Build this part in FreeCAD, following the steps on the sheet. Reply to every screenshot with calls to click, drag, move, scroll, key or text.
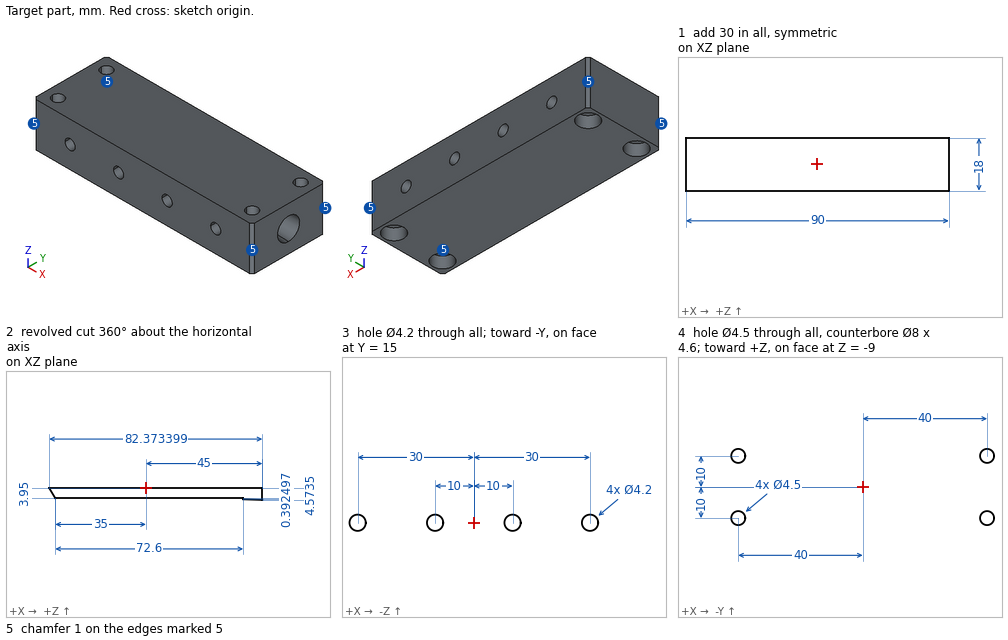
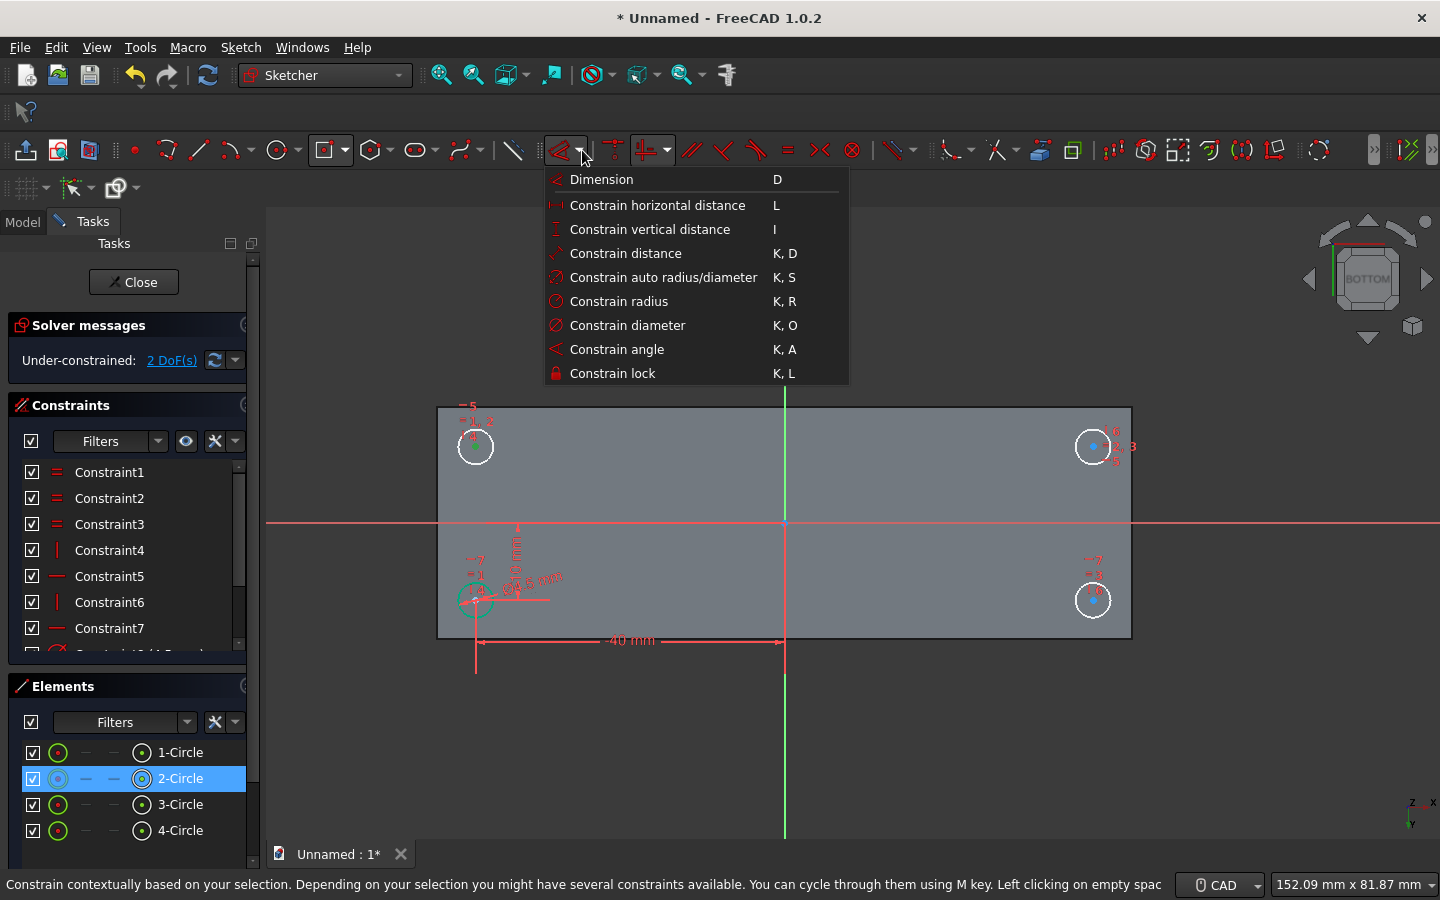
click(697, 229)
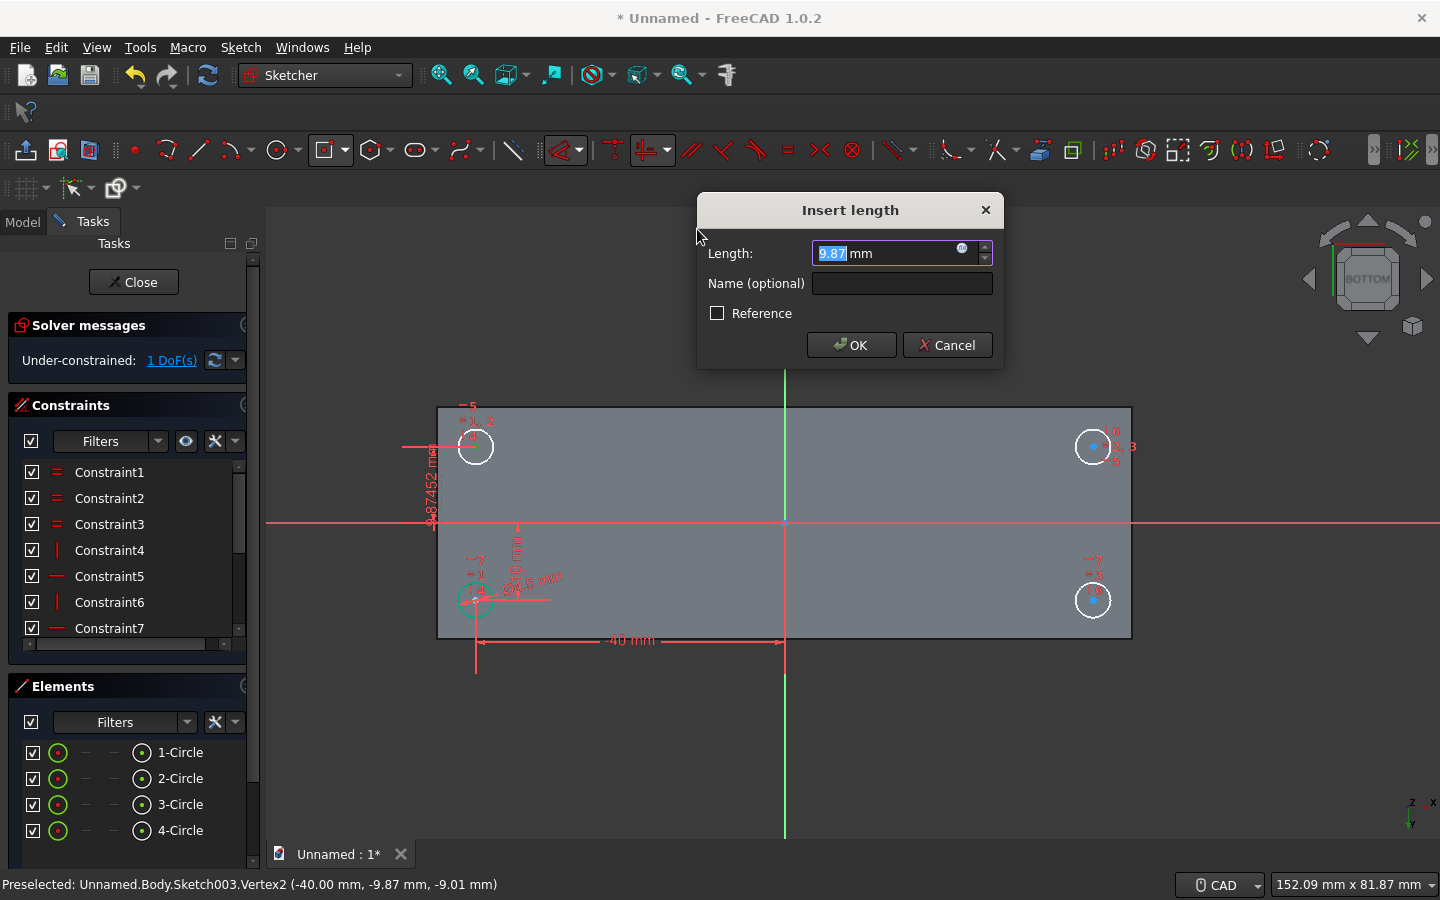
text(10)
key(Return)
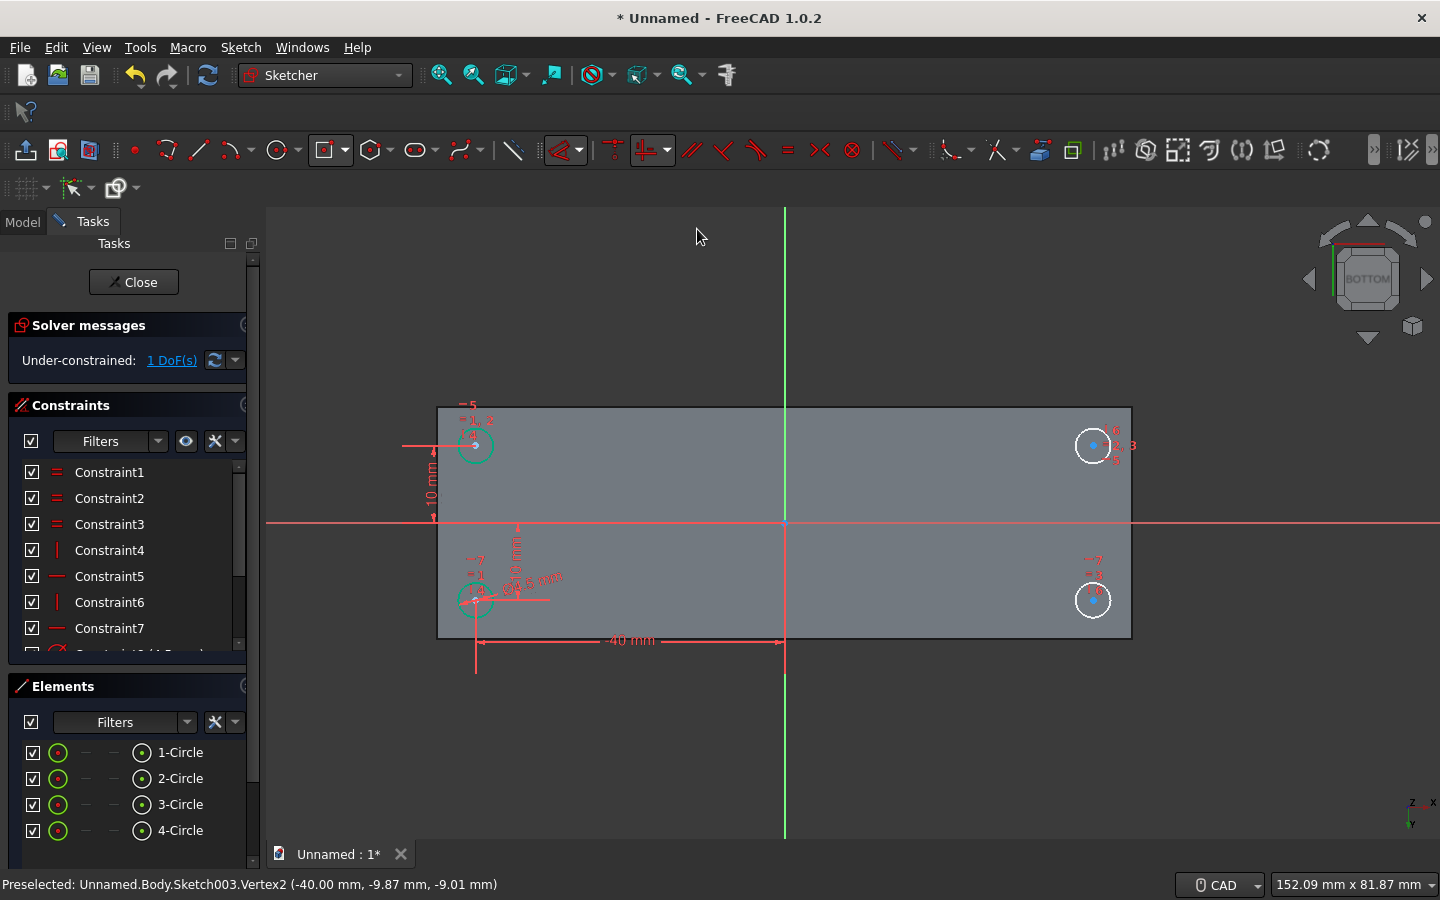
click(1093, 446)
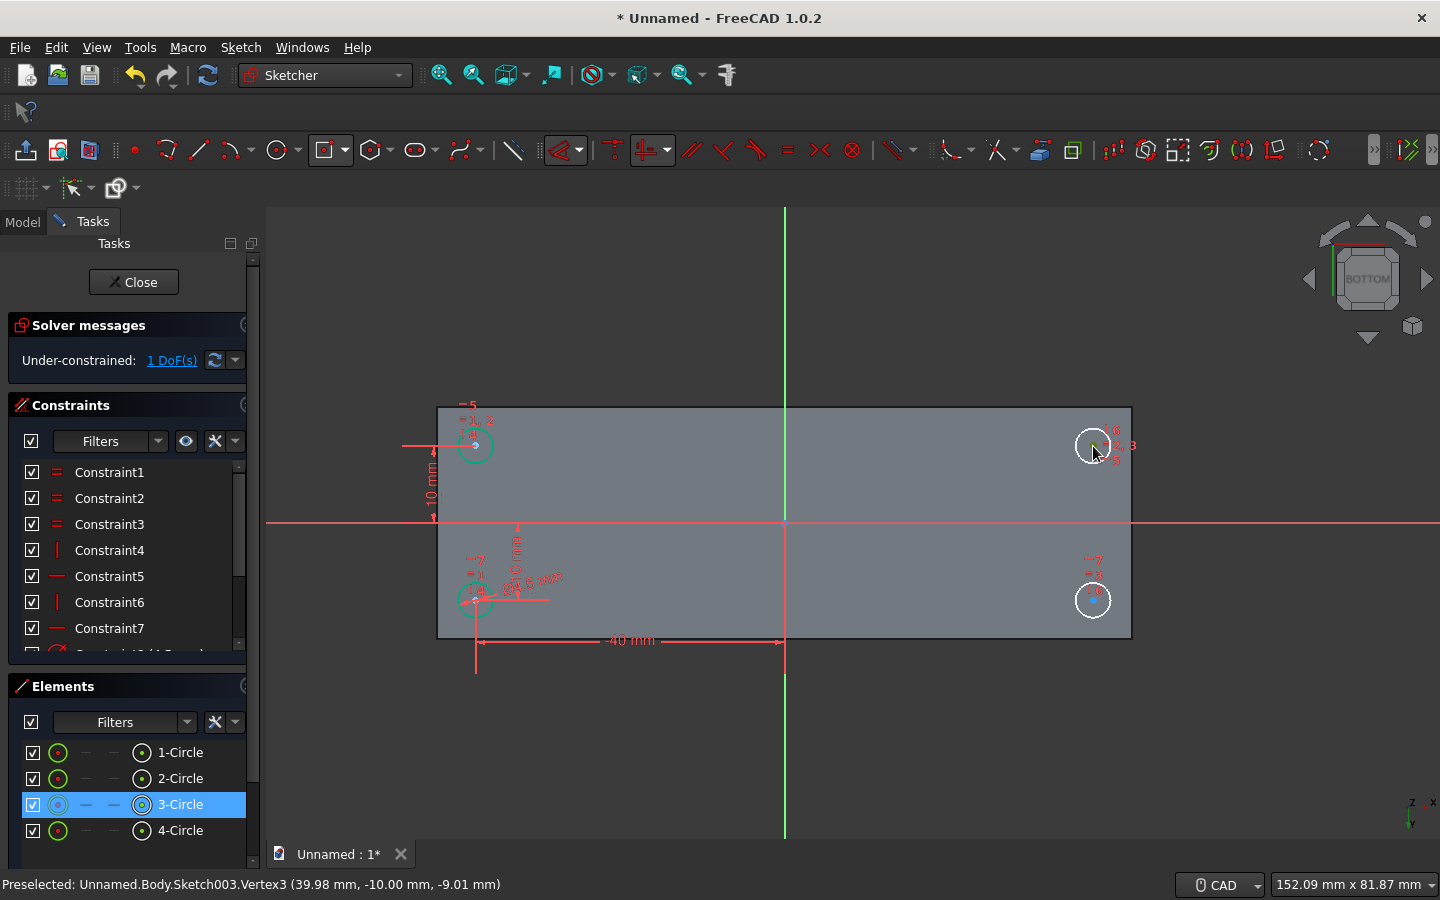
key(l)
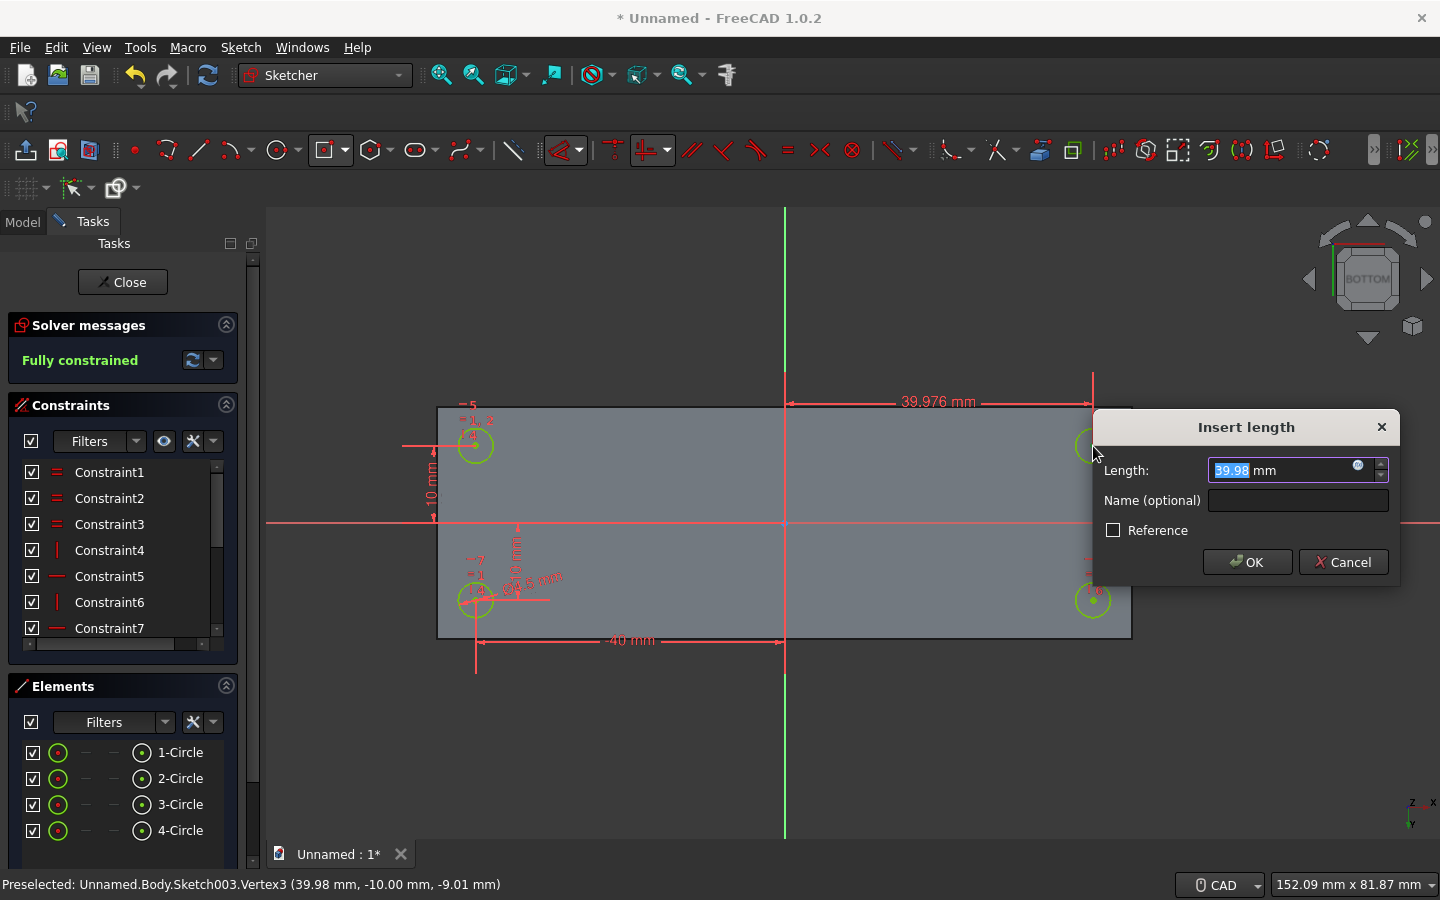
text(40)
key(Return)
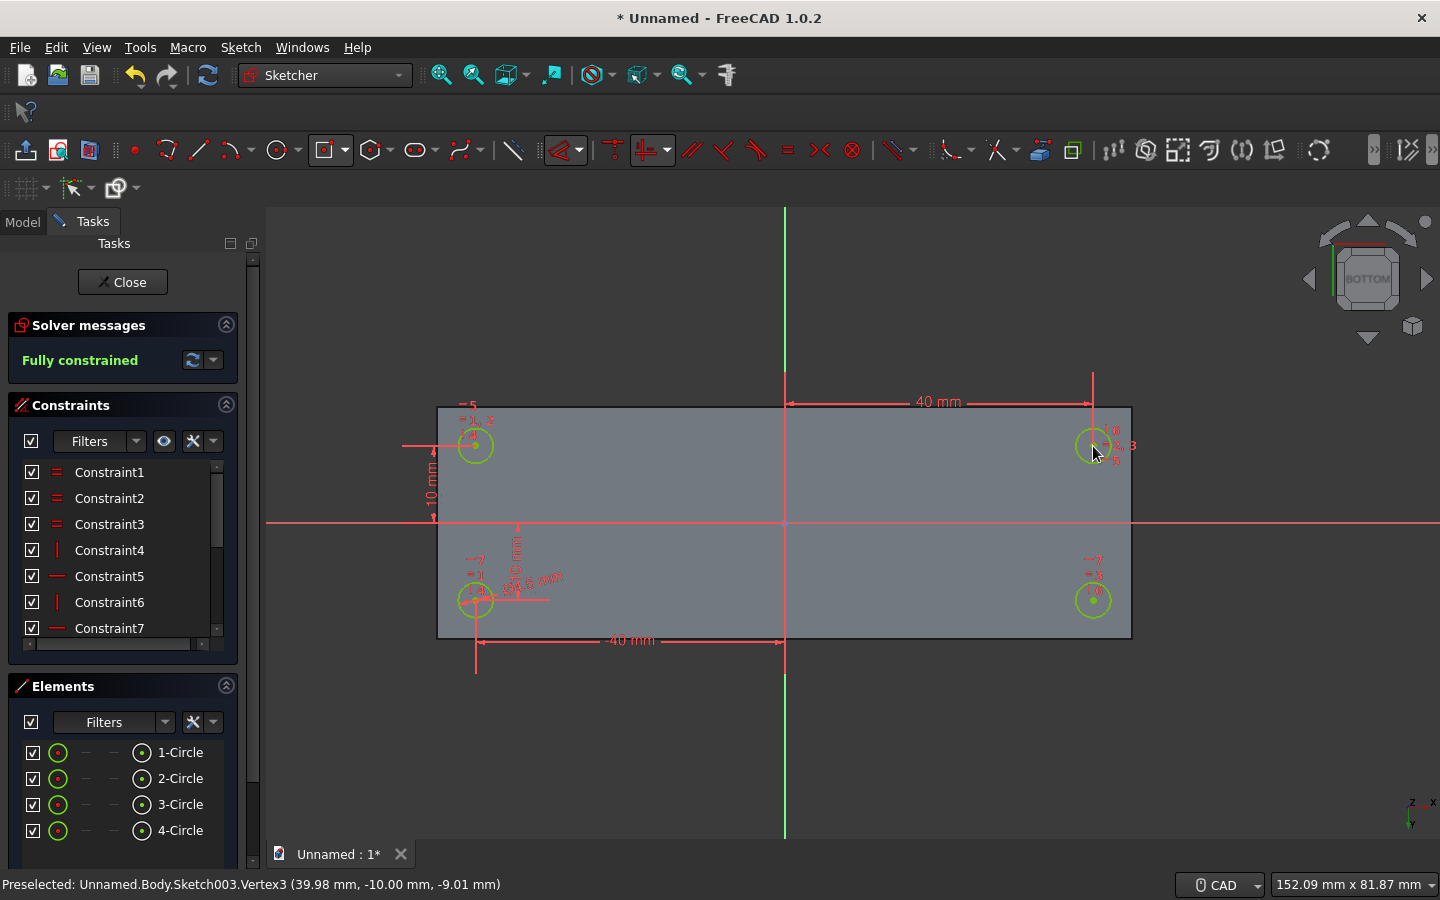
click(123, 282)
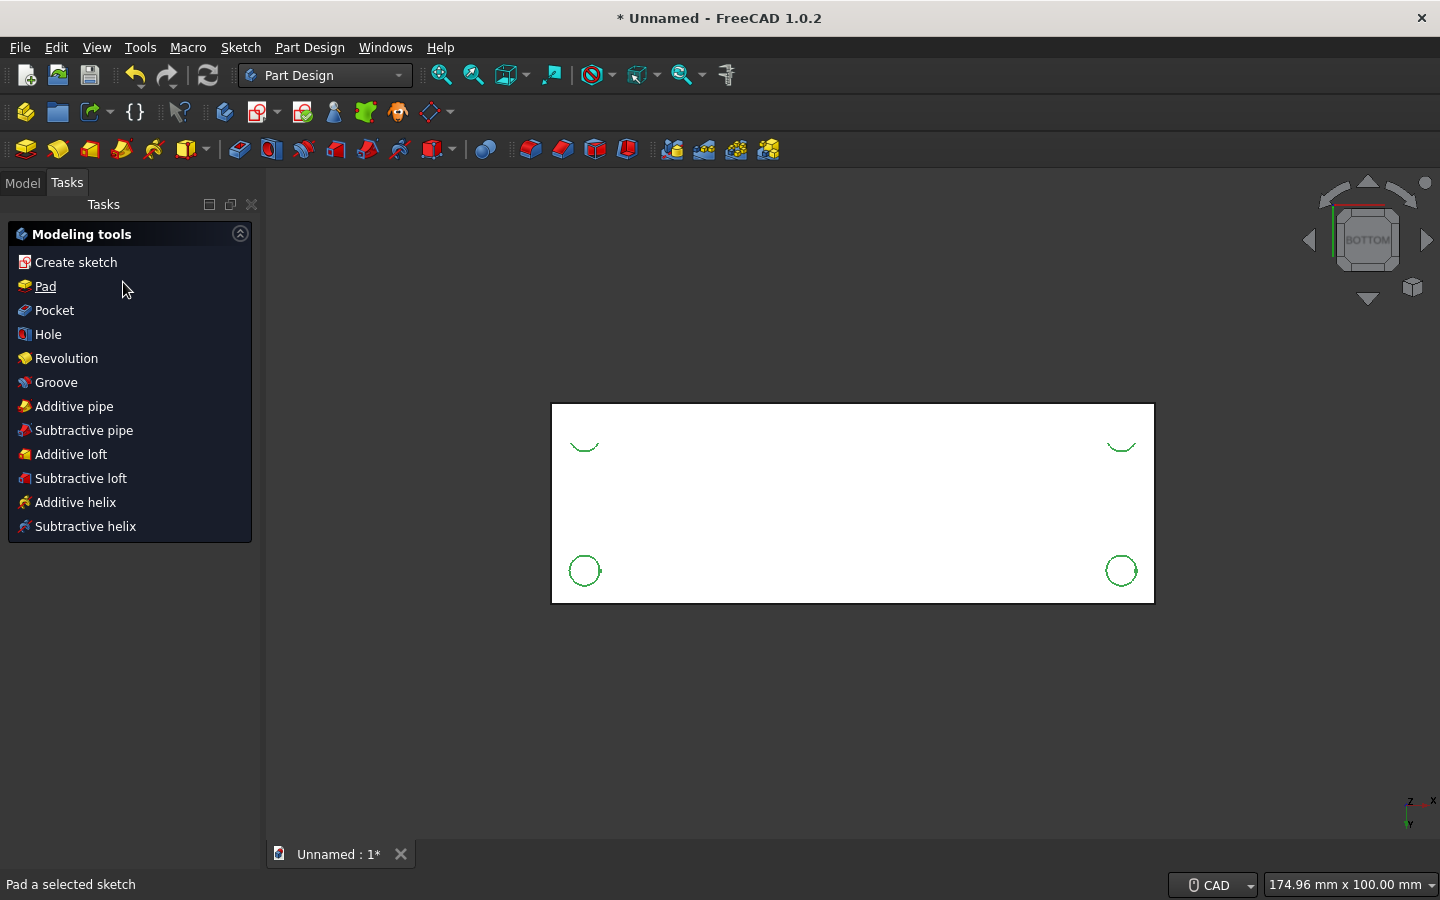
click(272, 150)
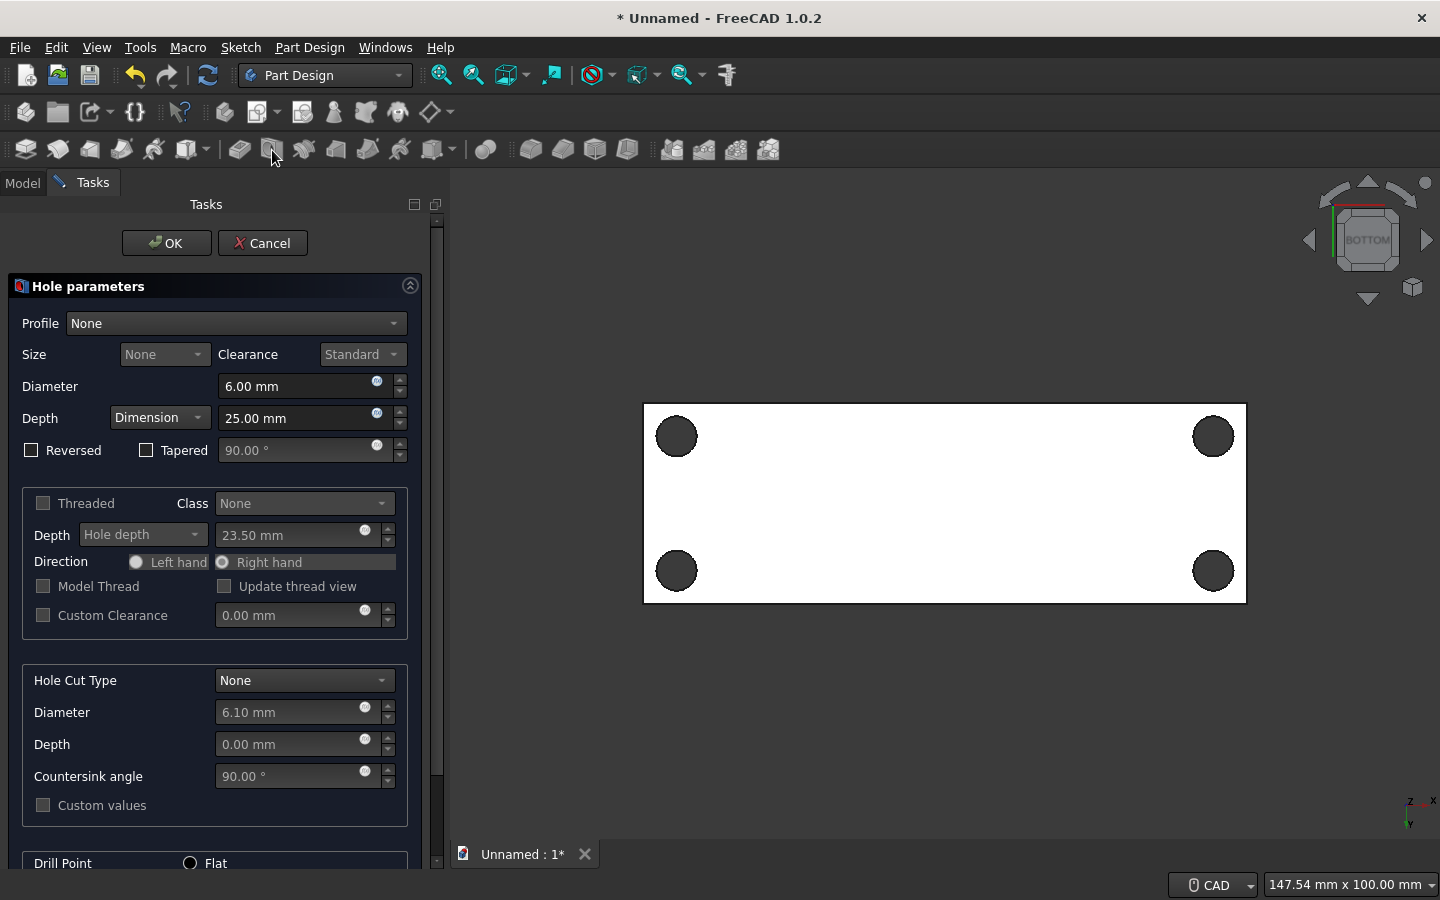
triple_click(305, 386)